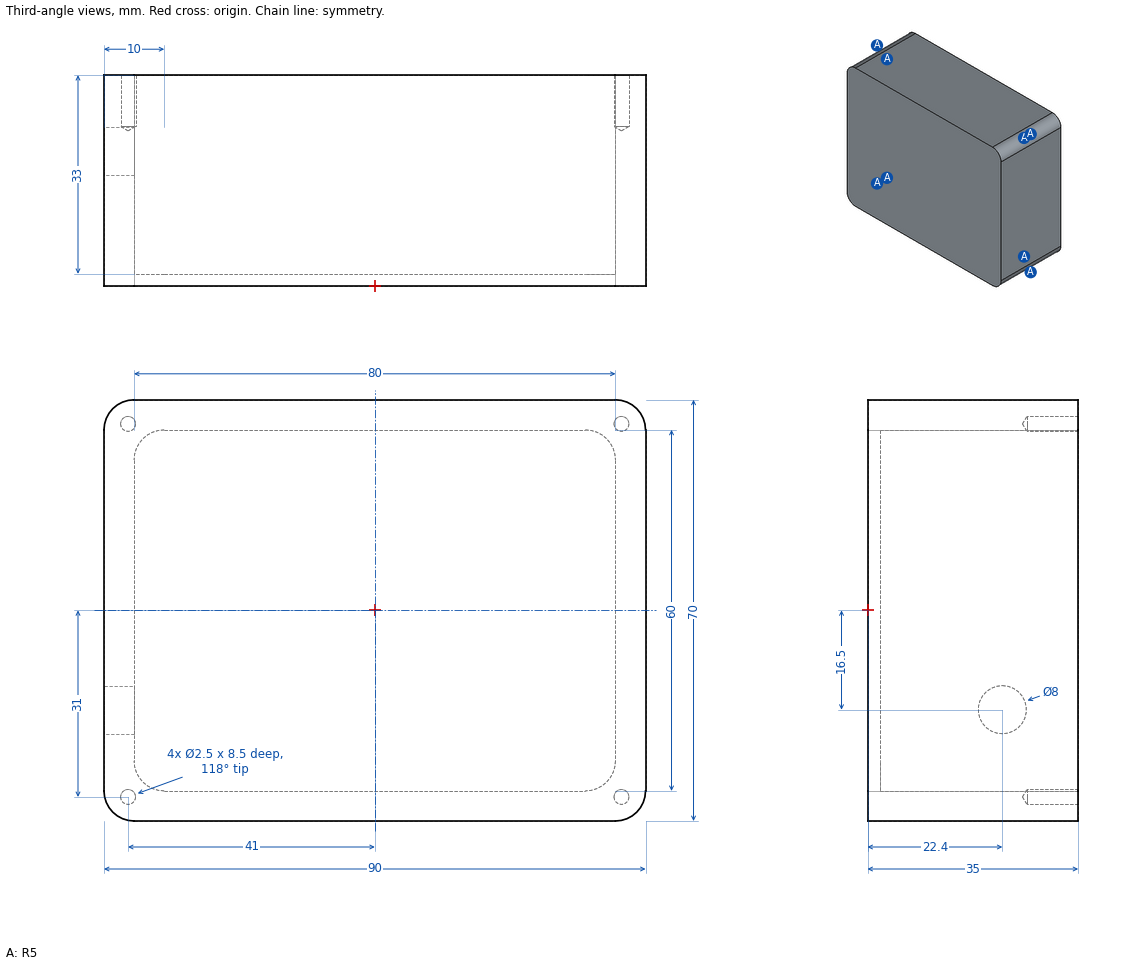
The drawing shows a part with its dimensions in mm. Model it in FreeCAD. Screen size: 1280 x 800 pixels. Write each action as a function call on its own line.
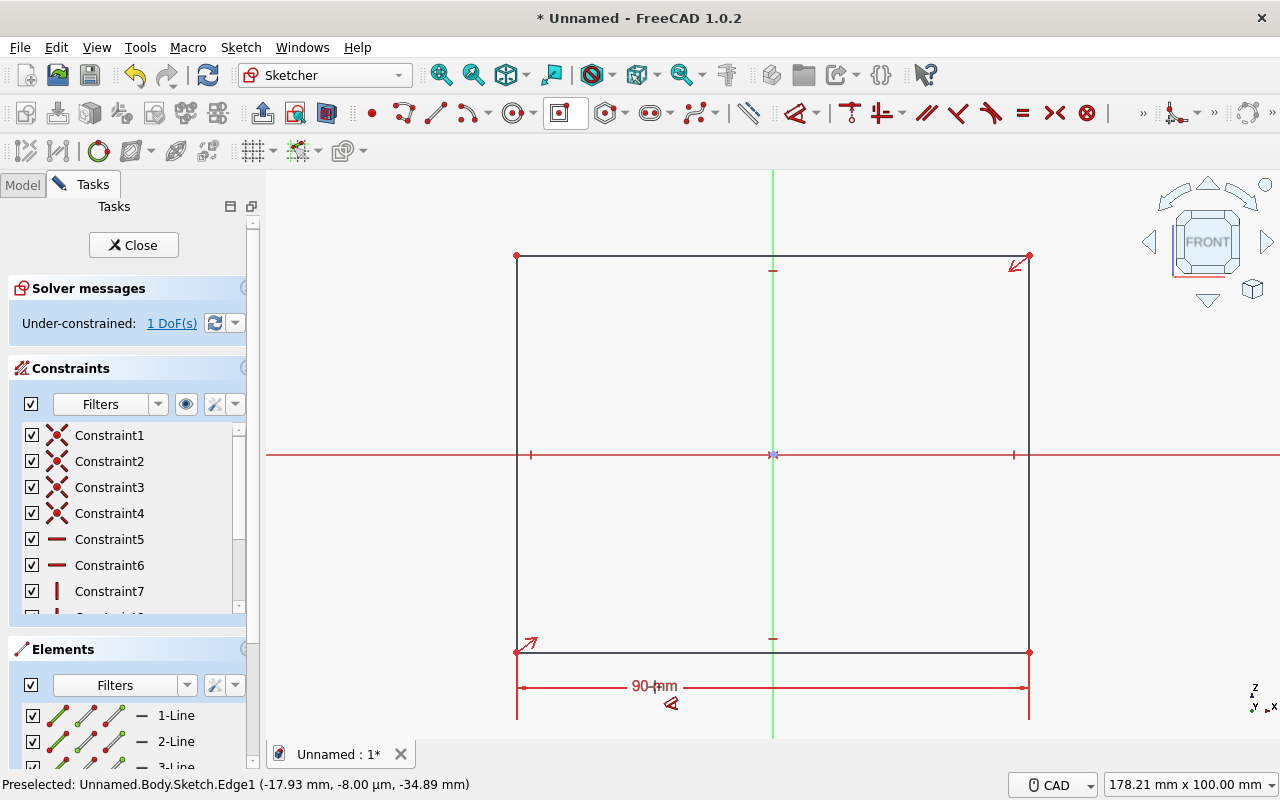
click(1029, 534)
click(1063, 363)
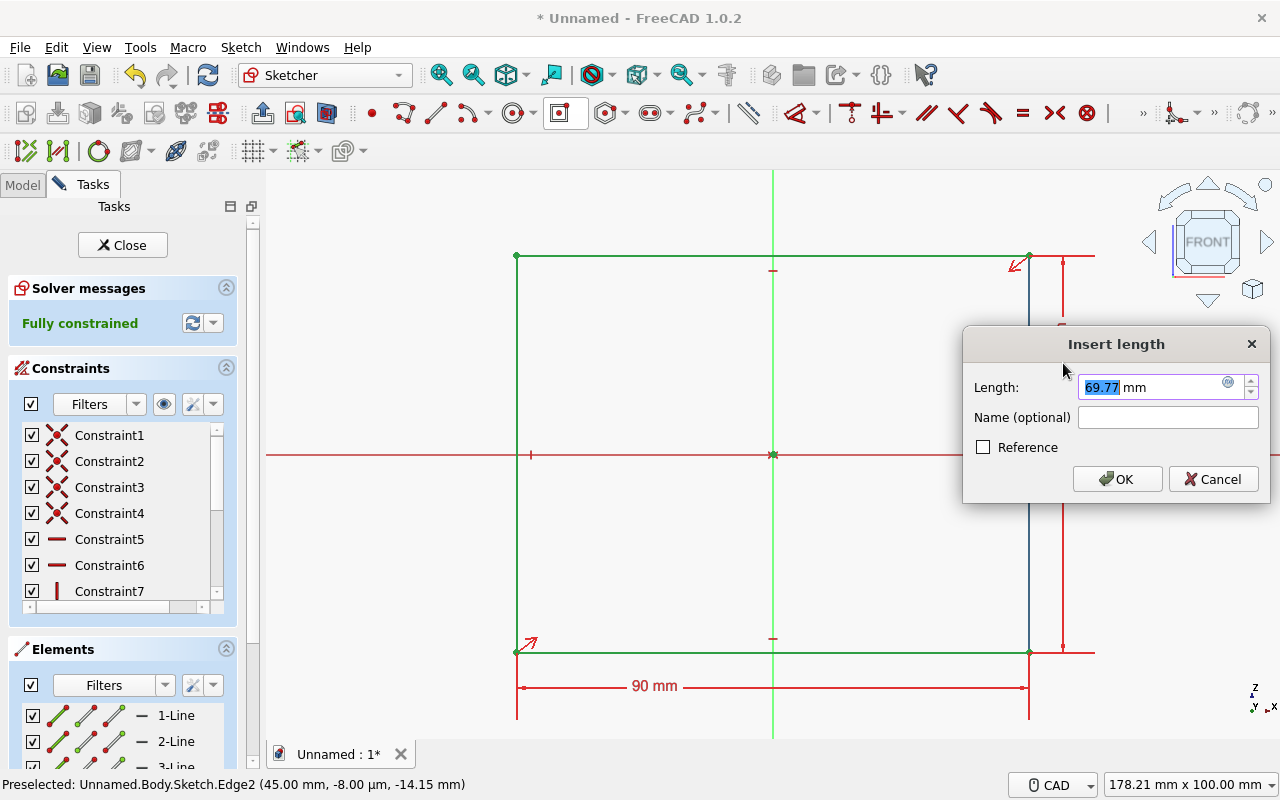
text(70)
key(Return)
key(Escape)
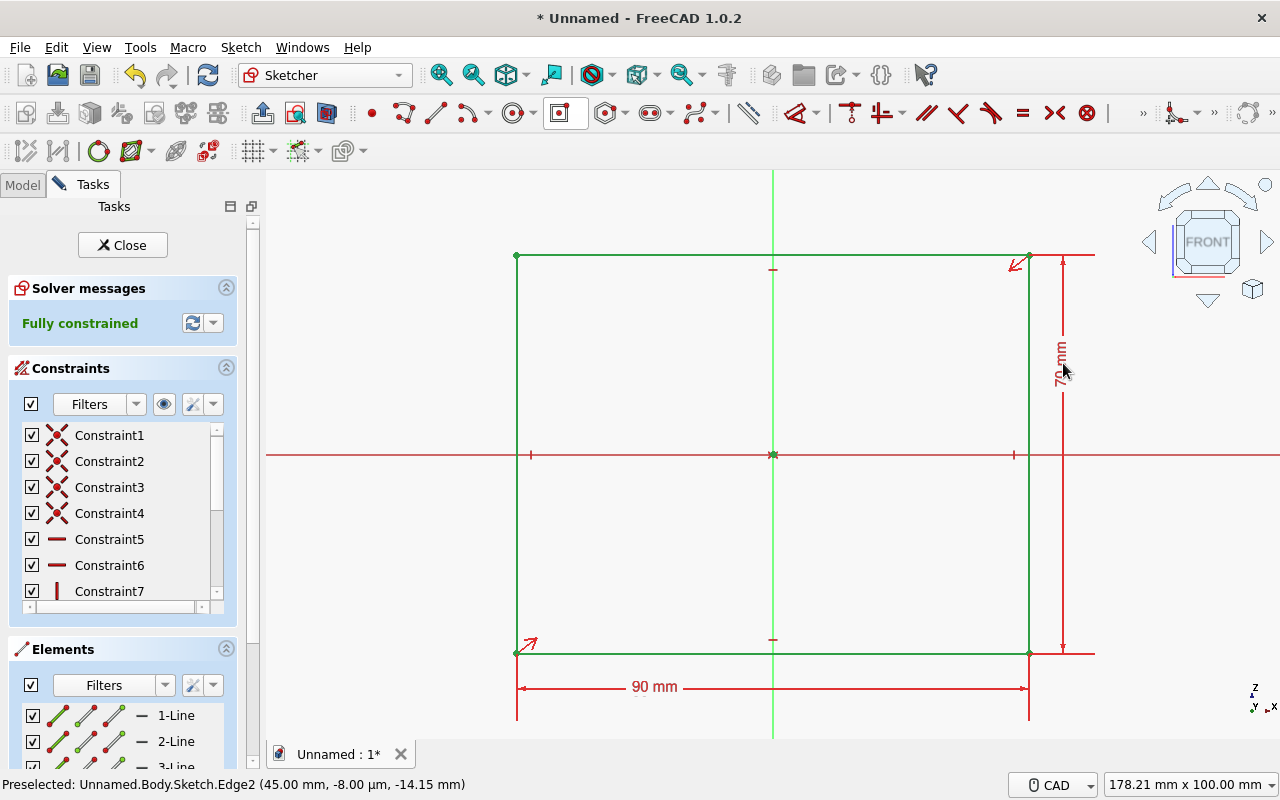
click(123, 245)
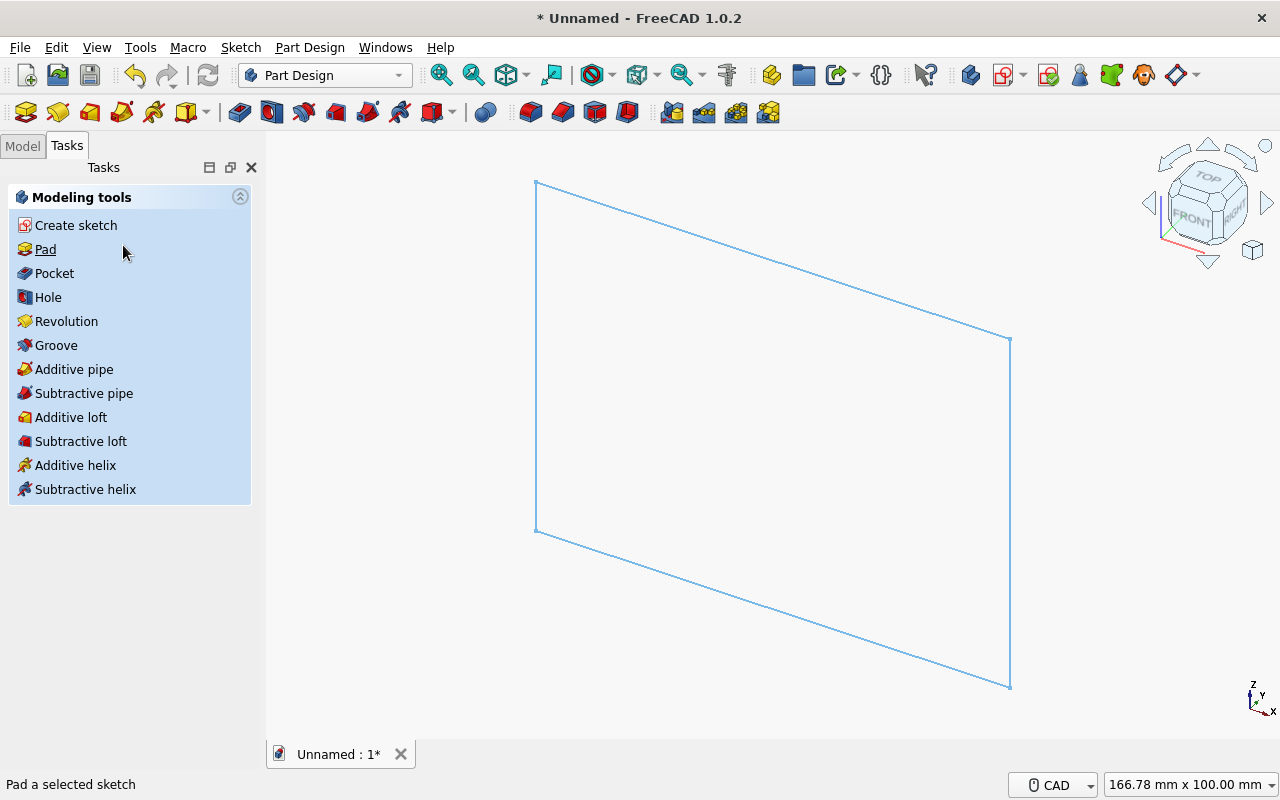
click(26, 112)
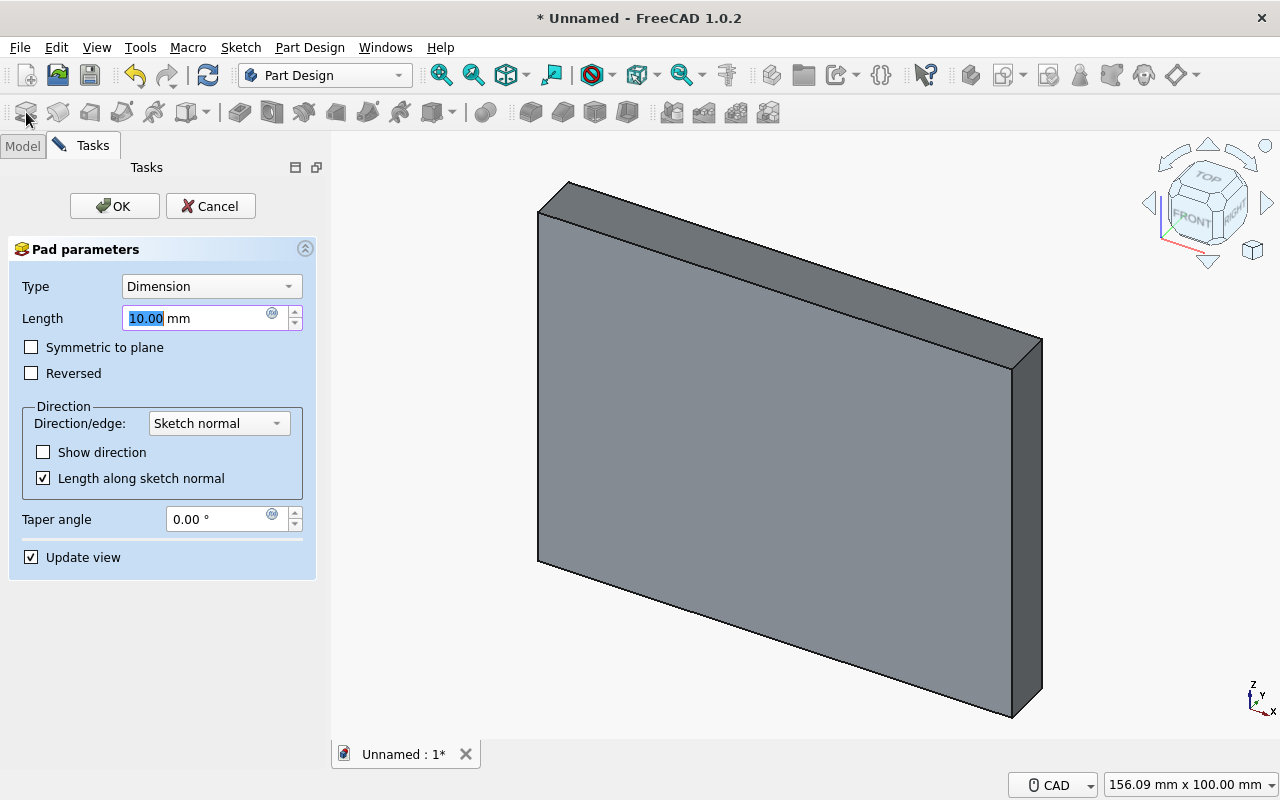
text(35)
key(Tab)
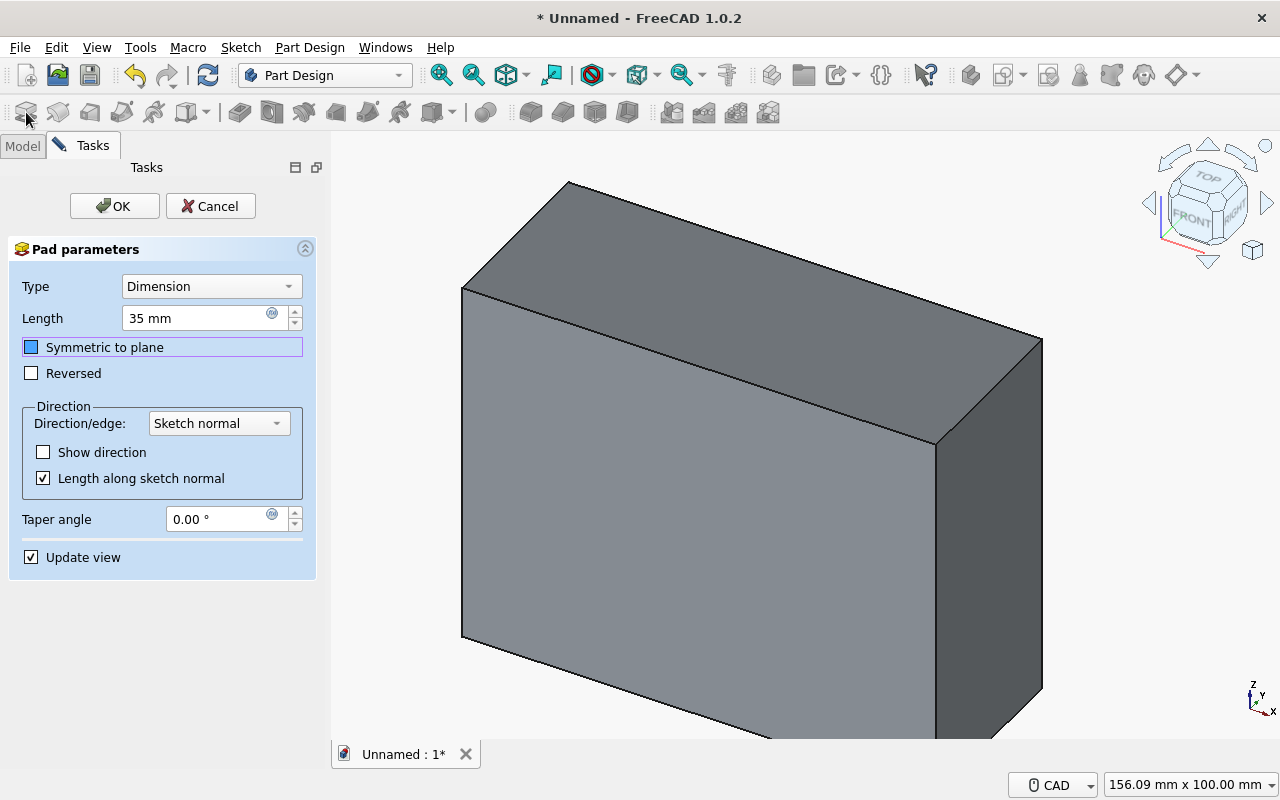
click(30, 373)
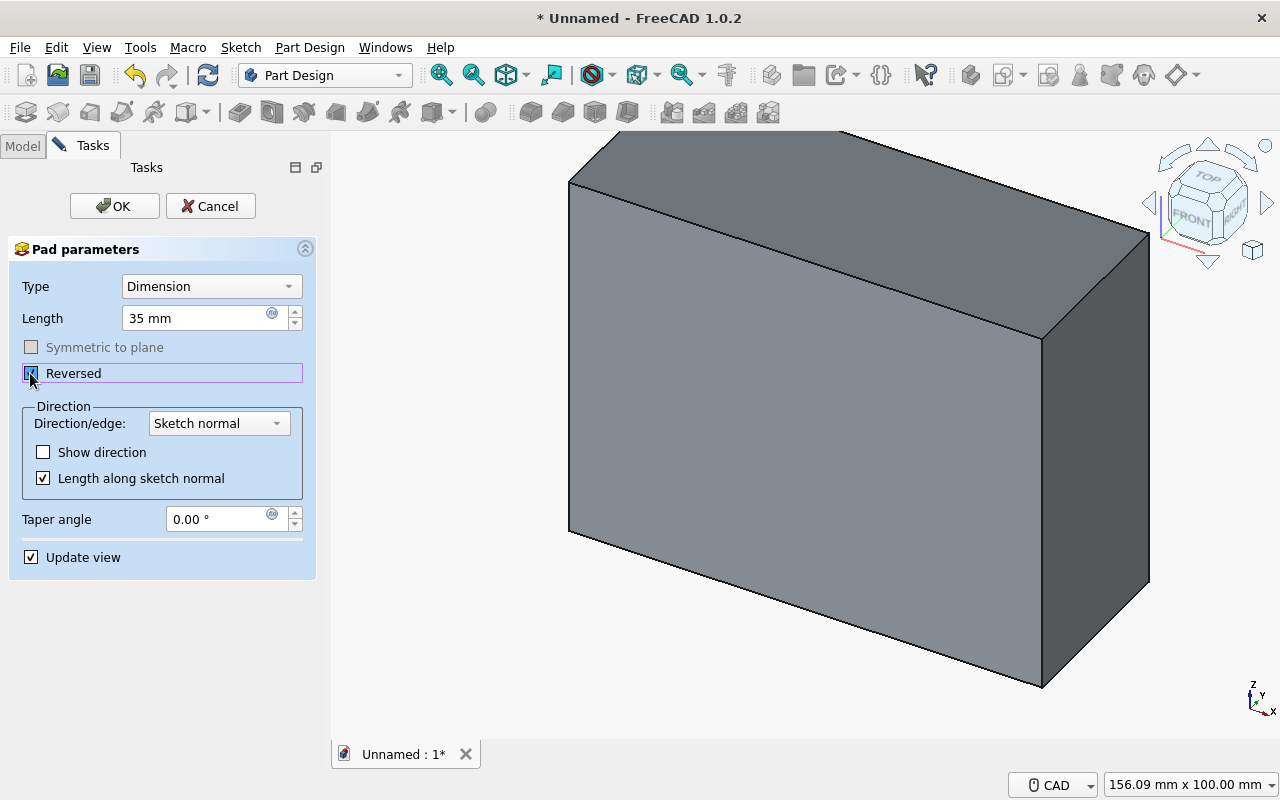
click(115, 206)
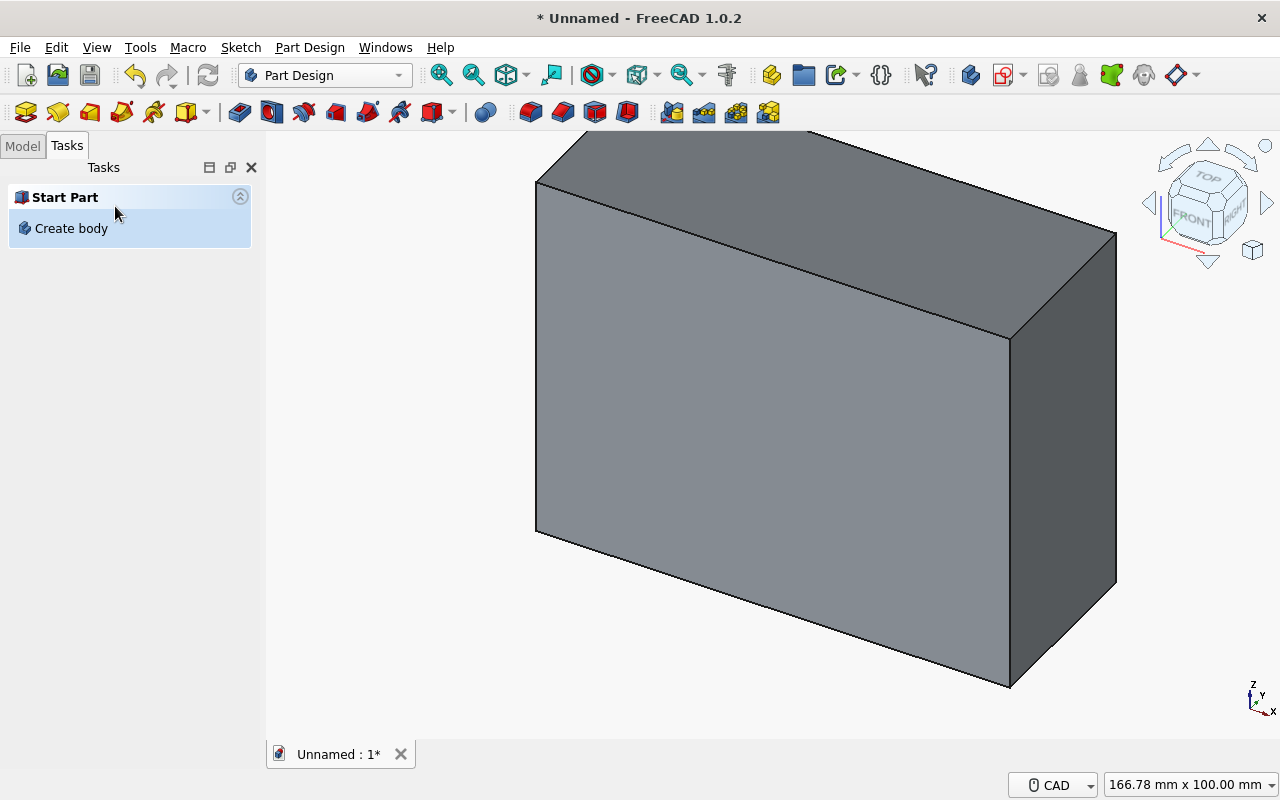
click(442, 76)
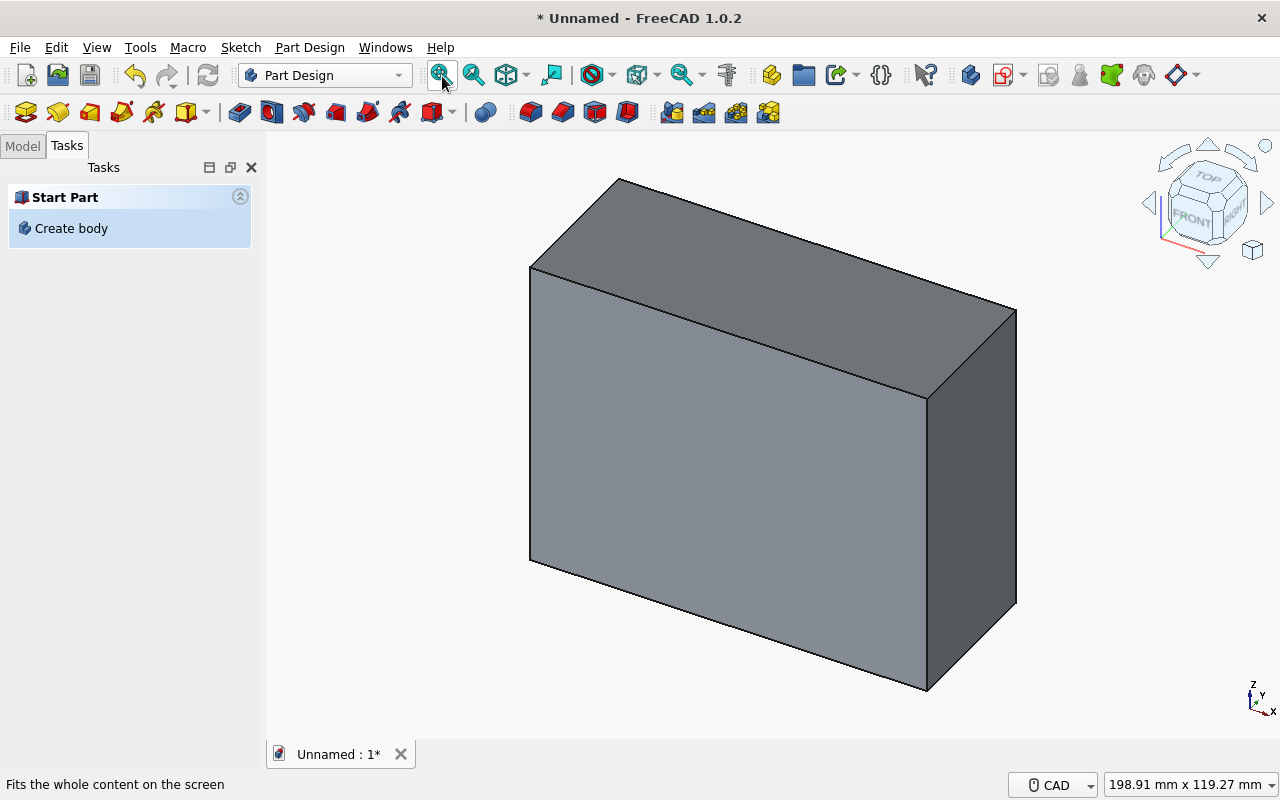
key(4)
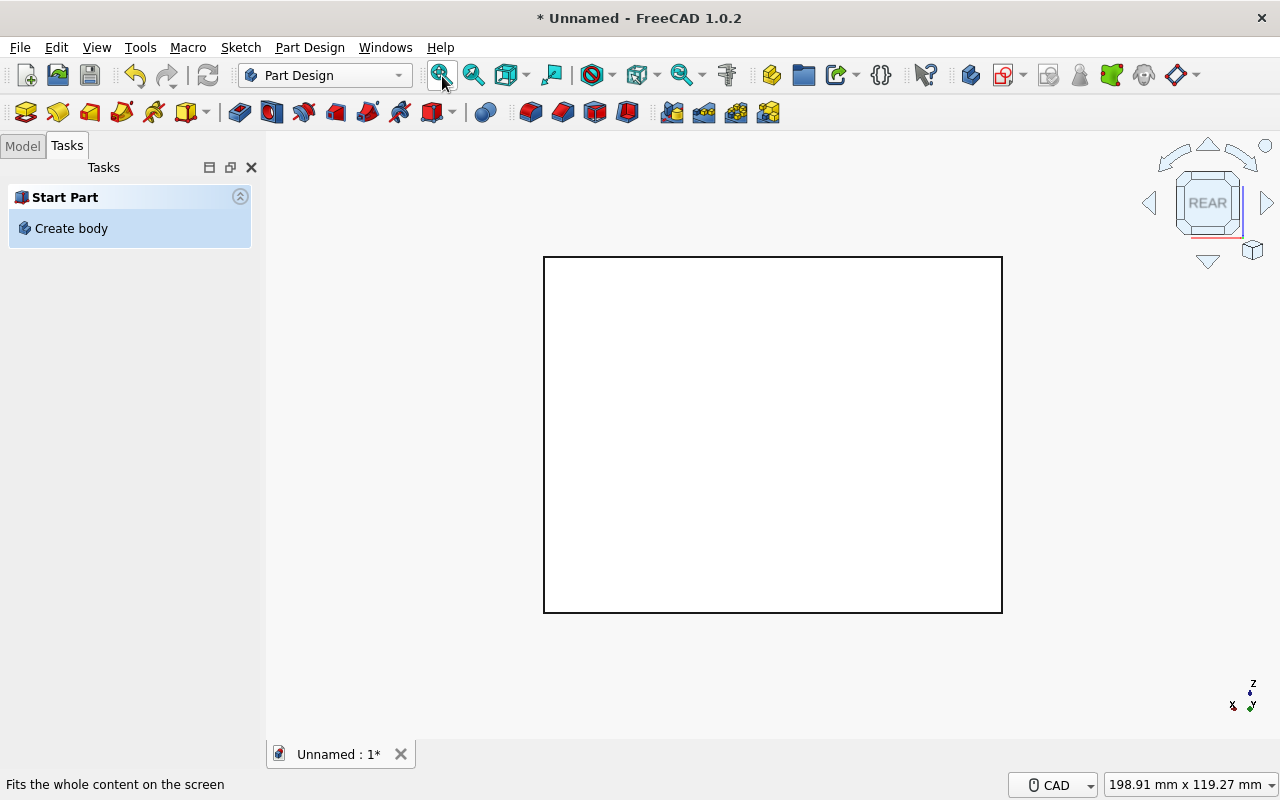
click(773, 434)